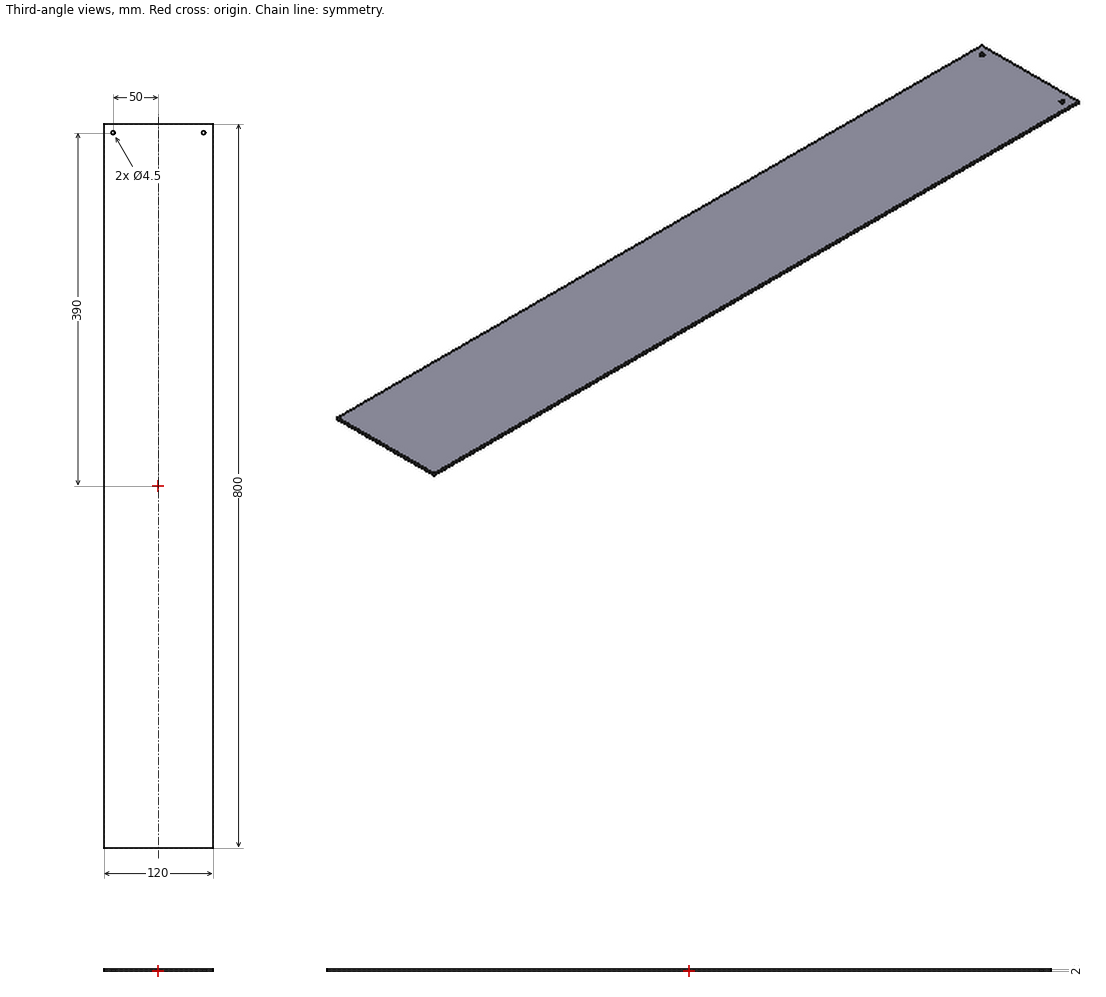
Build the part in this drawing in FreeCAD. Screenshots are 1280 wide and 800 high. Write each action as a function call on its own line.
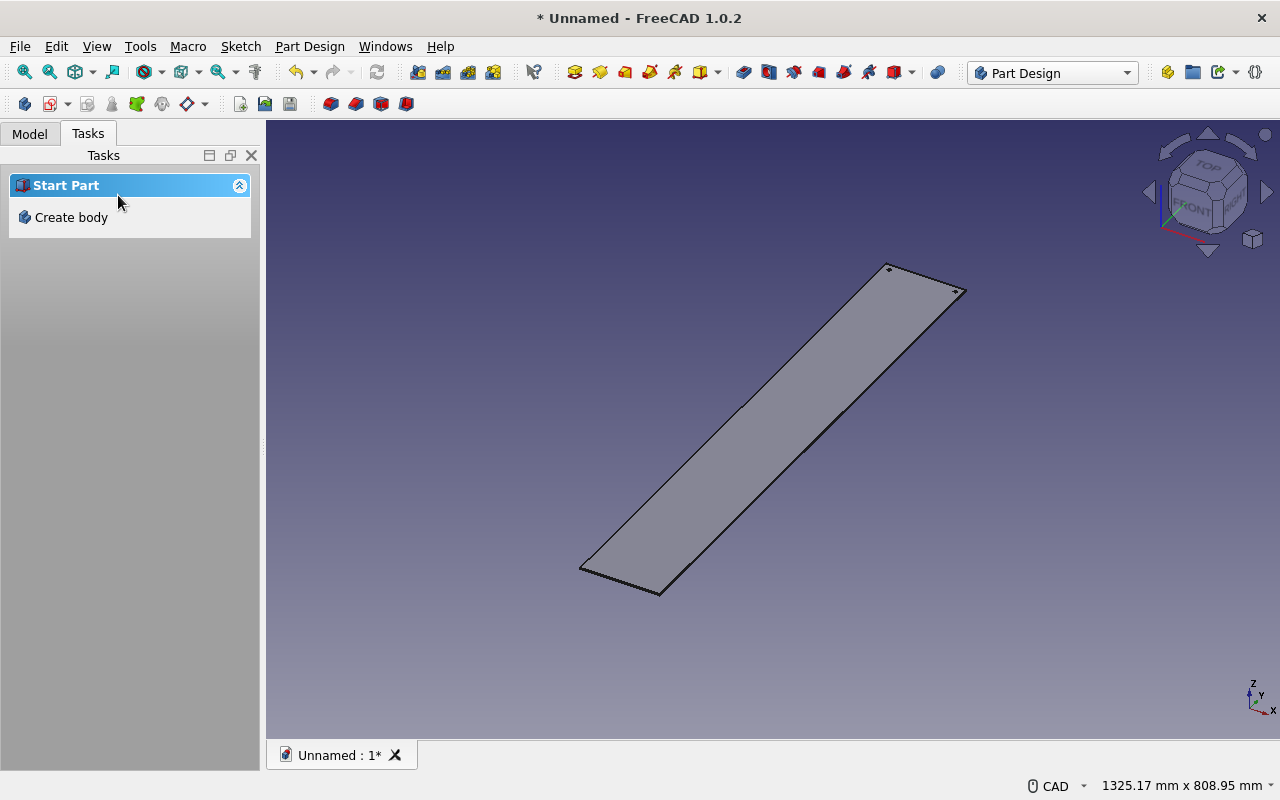
key(0)